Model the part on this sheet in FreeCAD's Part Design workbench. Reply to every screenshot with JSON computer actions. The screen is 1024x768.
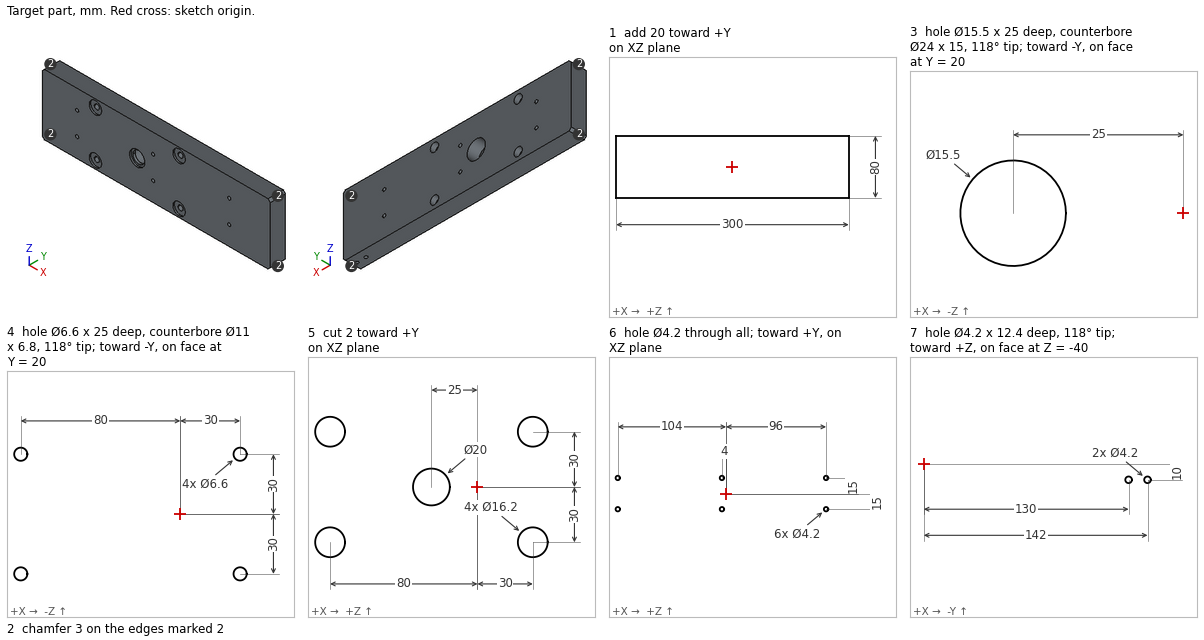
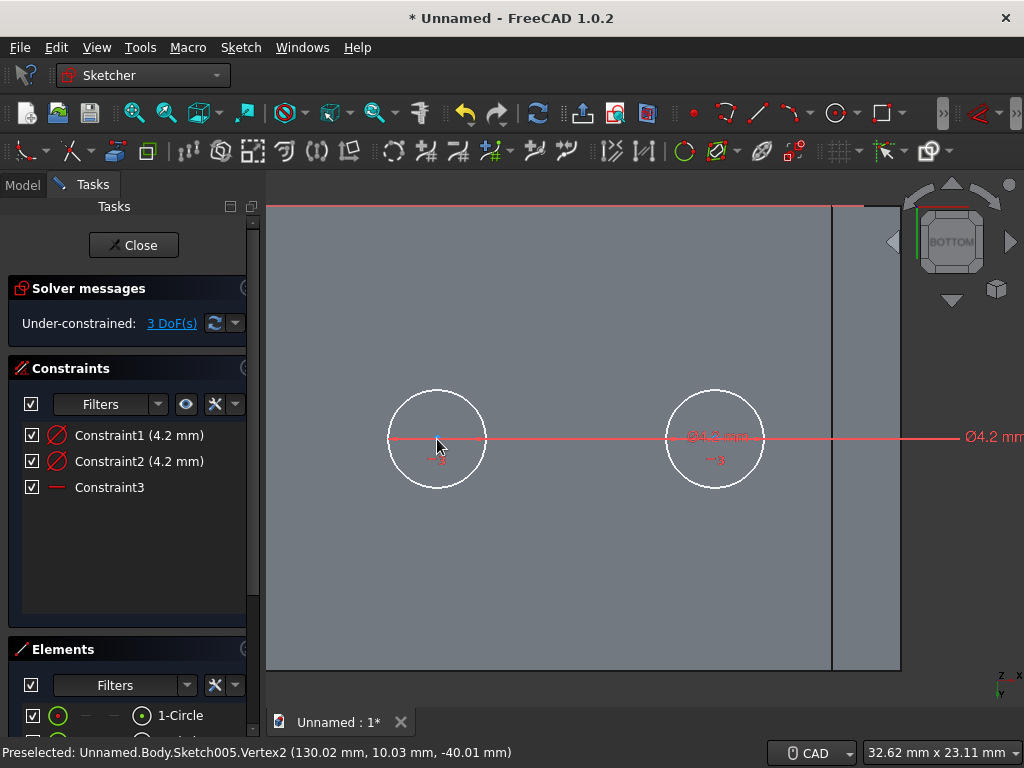
{"action": "left_click", "coordinate": [978, 114]}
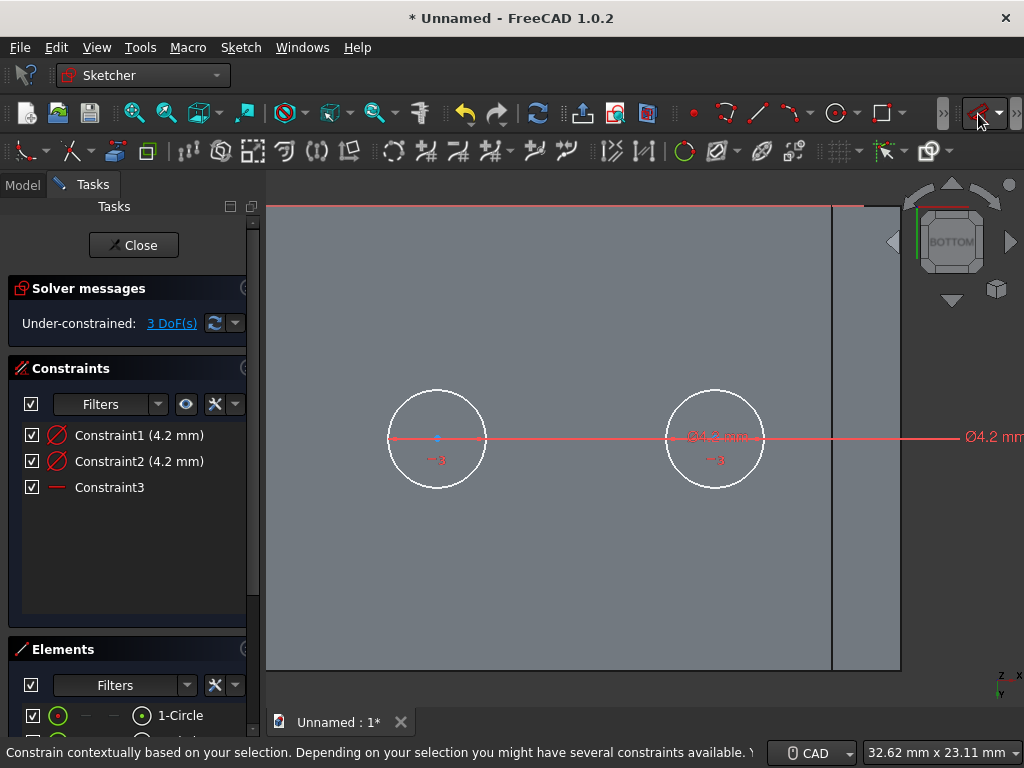
{"action": "left_click", "coordinate": [715, 439]}
{"action": "left_click", "coordinate": [749, 322]}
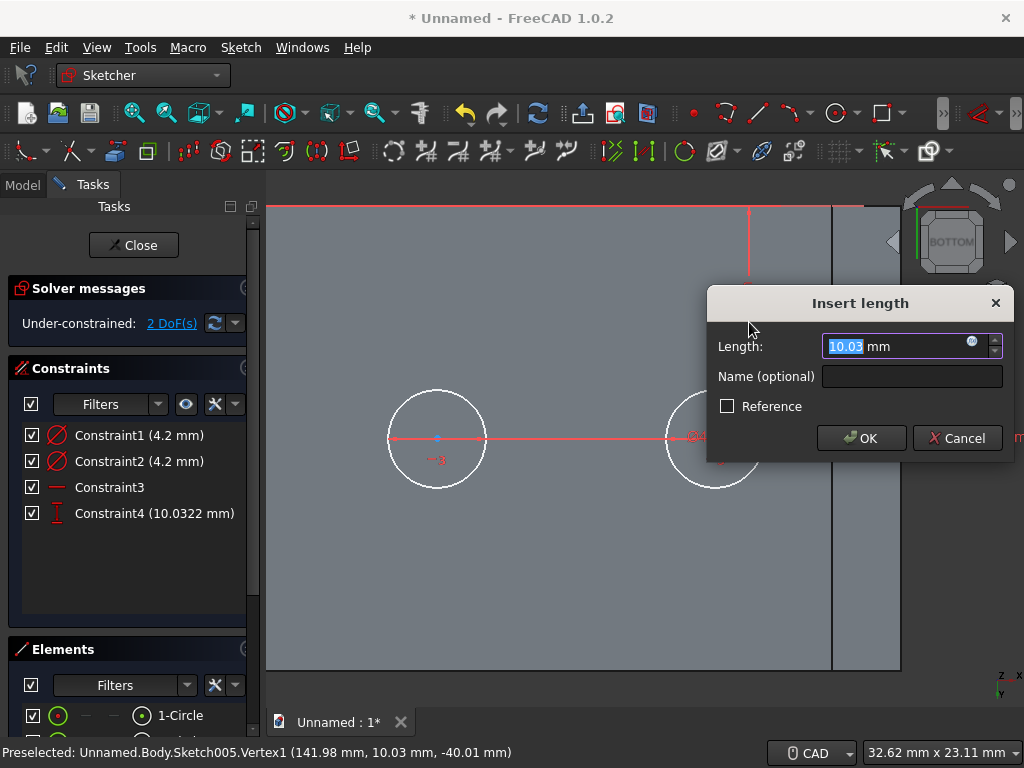
{"action": "type", "text": "10"}
{"action": "key", "text": "Return"}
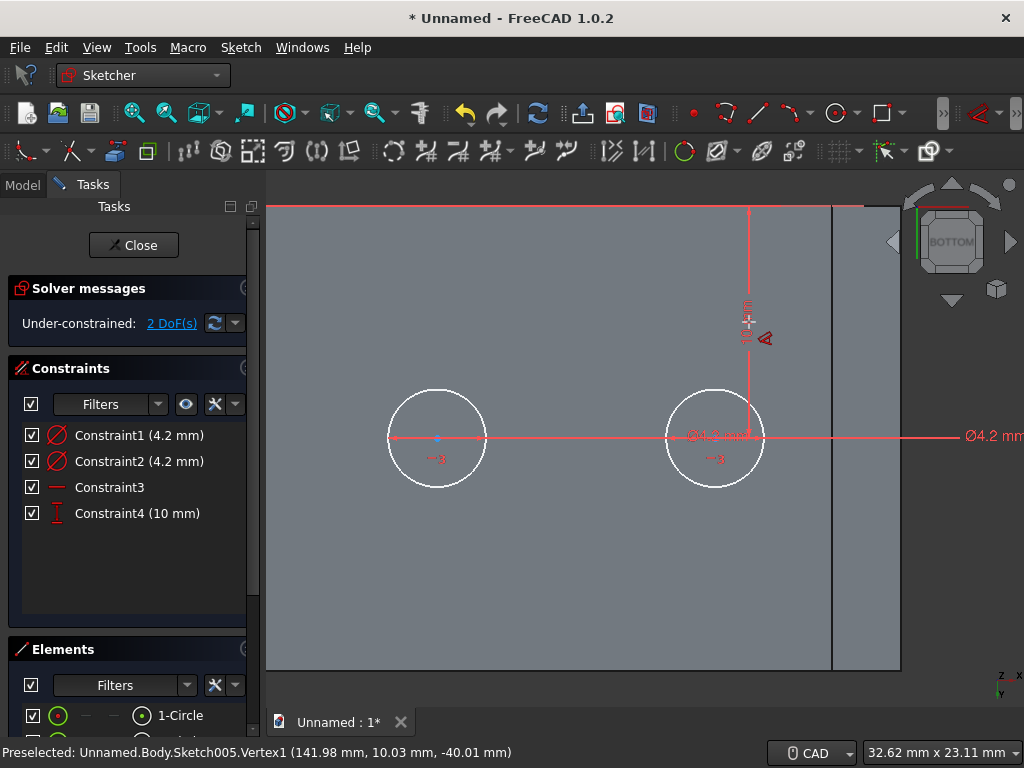
{"action": "left_click", "coordinate": [715, 438]}
{"action": "left_click", "coordinate": [504, 472]}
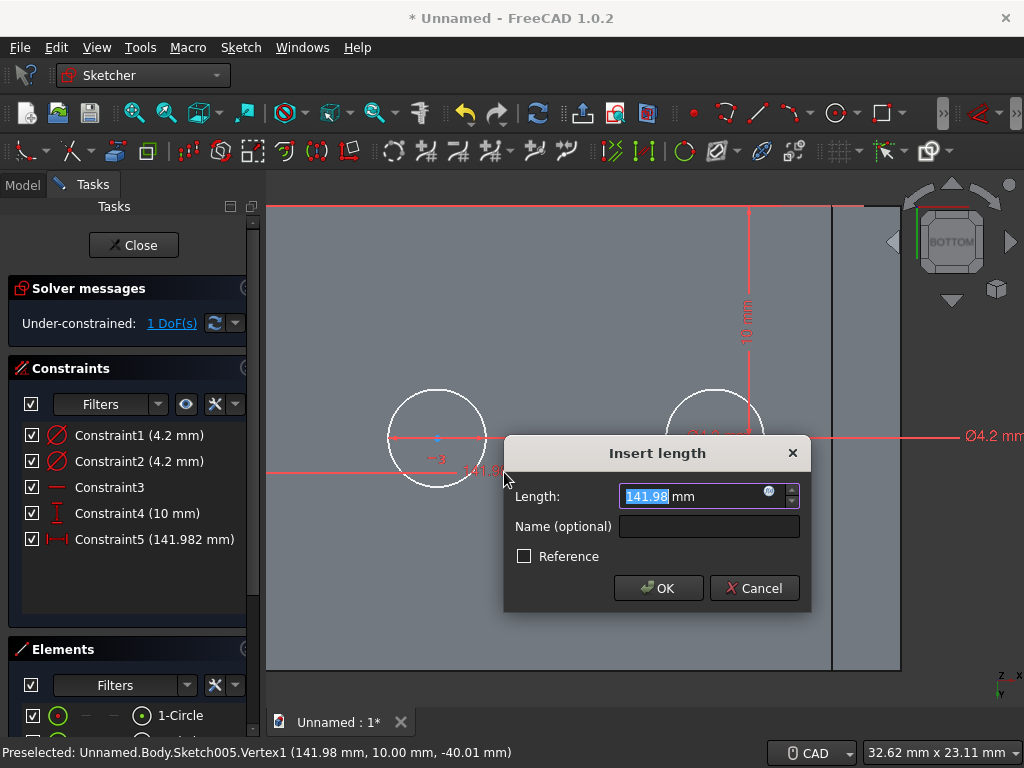
{"action": "type", "text": "142"}
{"action": "key", "text": "Return"}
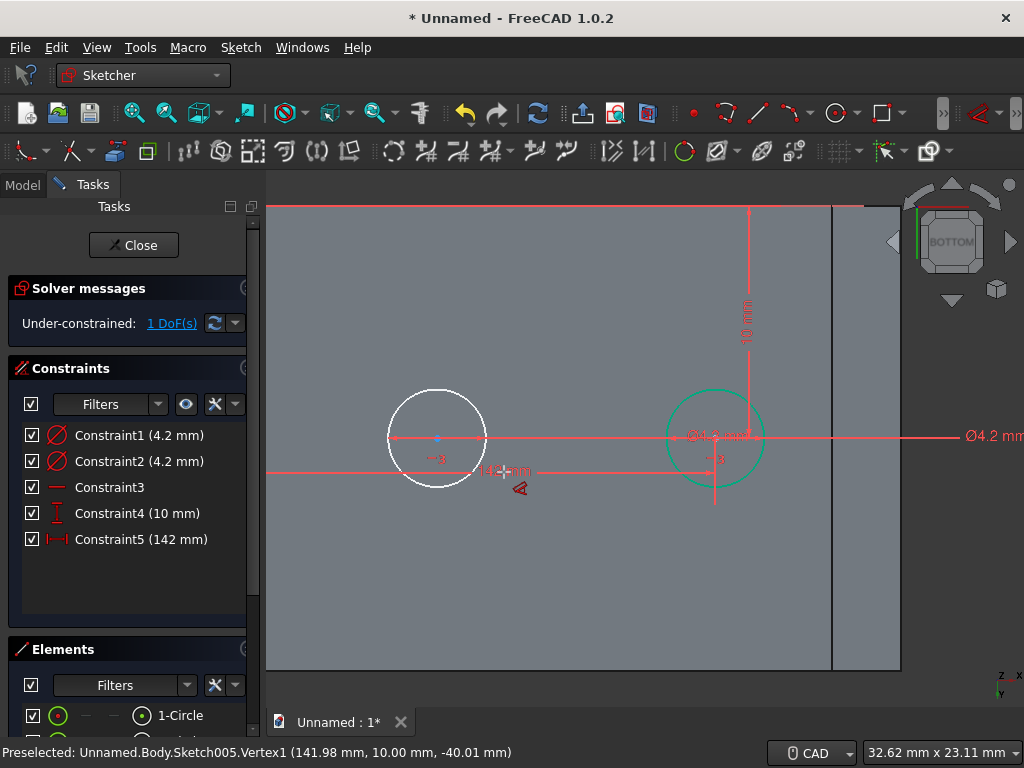
{"action": "left_click", "coordinate": [437, 438]}
{"action": "left_click", "coordinate": [365, 472]}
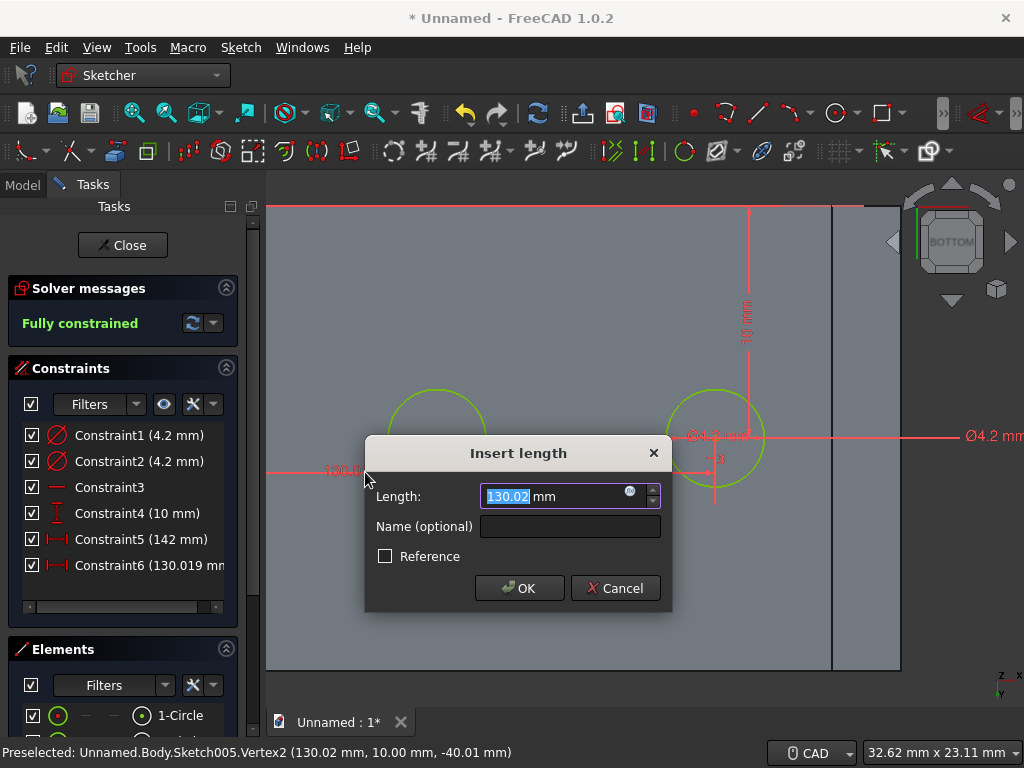
{"action": "type", "text": "130"}
{"action": "key", "text": "Return"}
{"action": "key", "text": "Escape"}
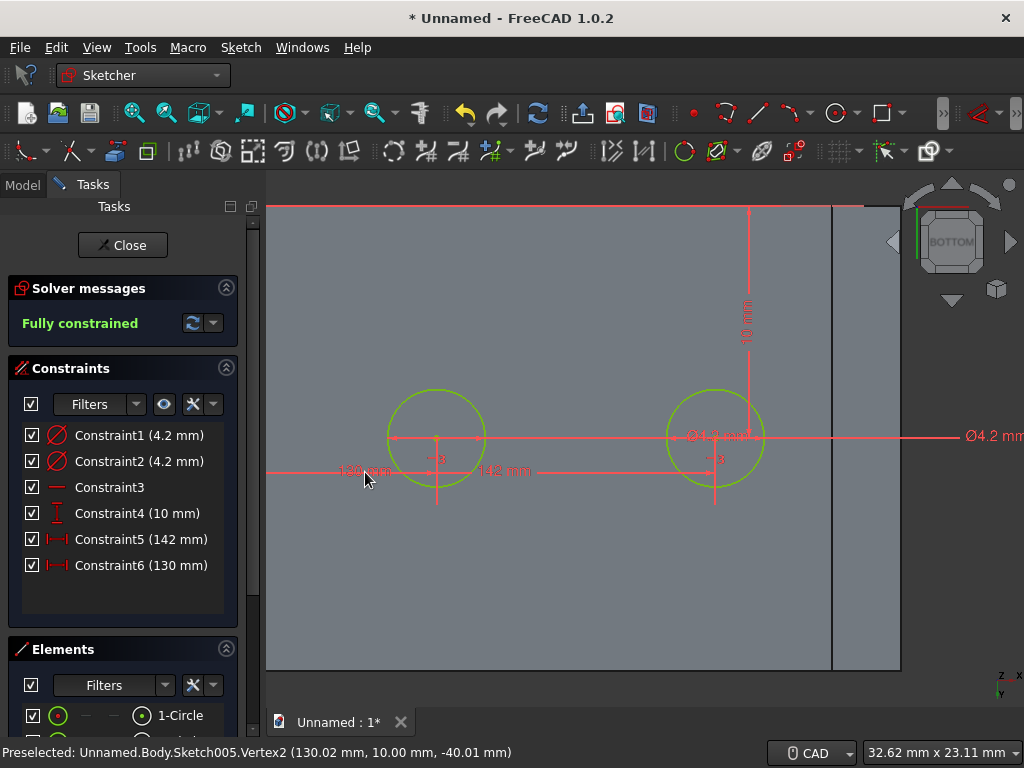
{"action": "left_click", "coordinate": [123, 245]}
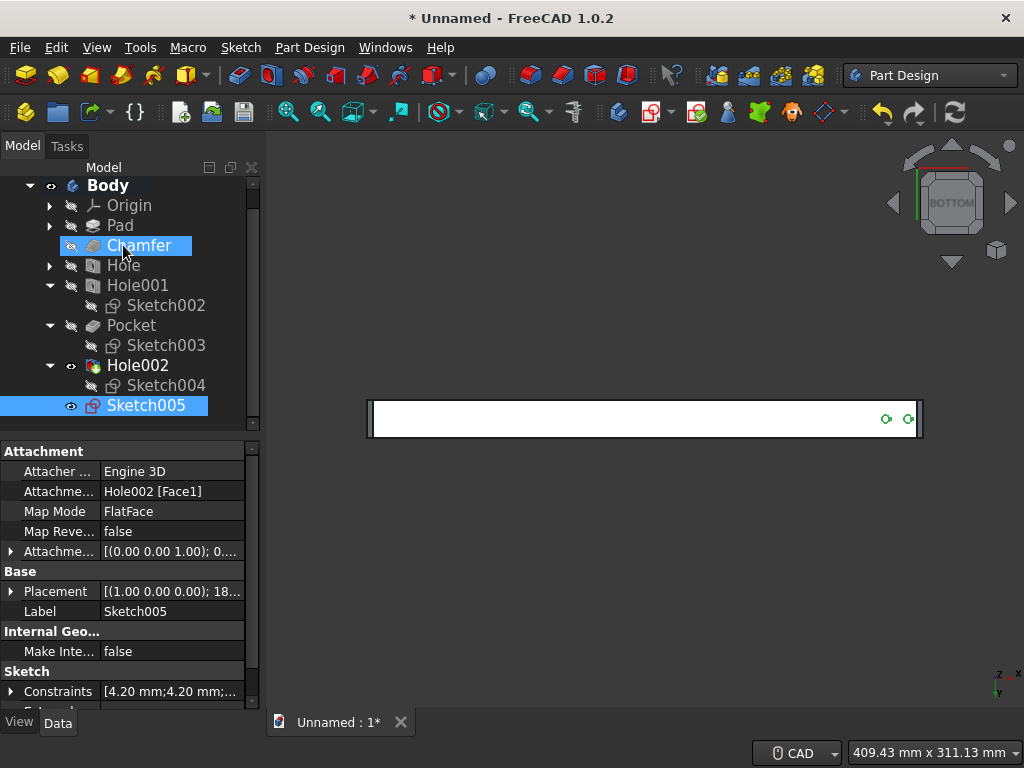
{"action": "left_click", "coordinate": [272, 76]}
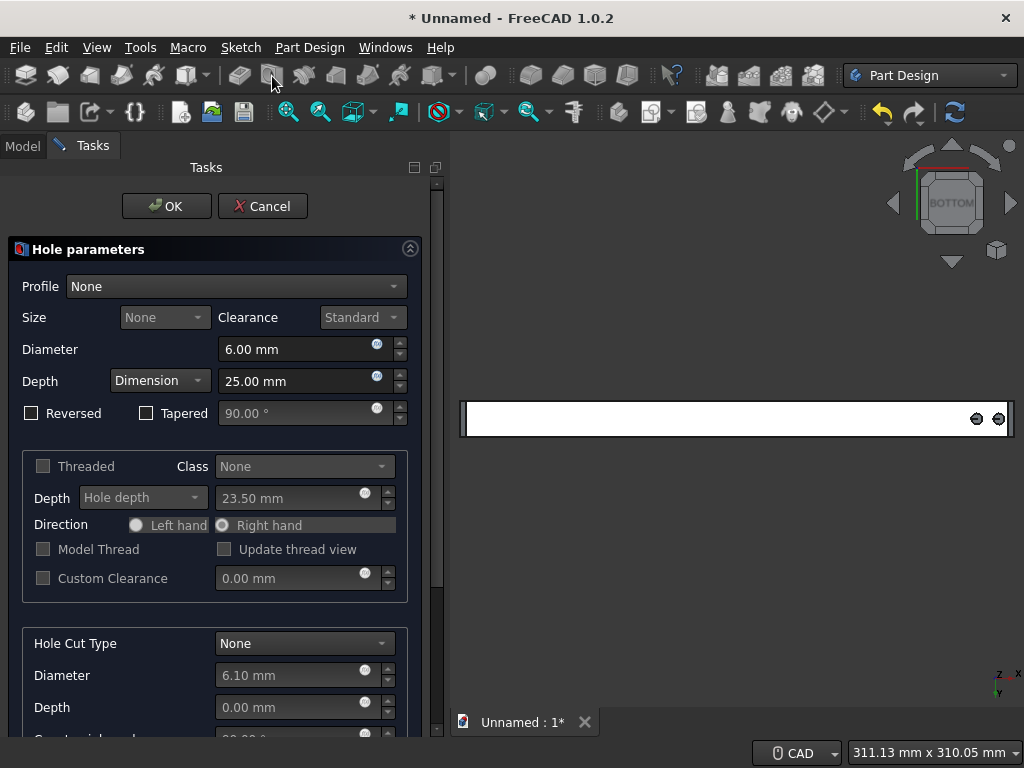
{"action": "triple_click", "coordinate": [305, 349]}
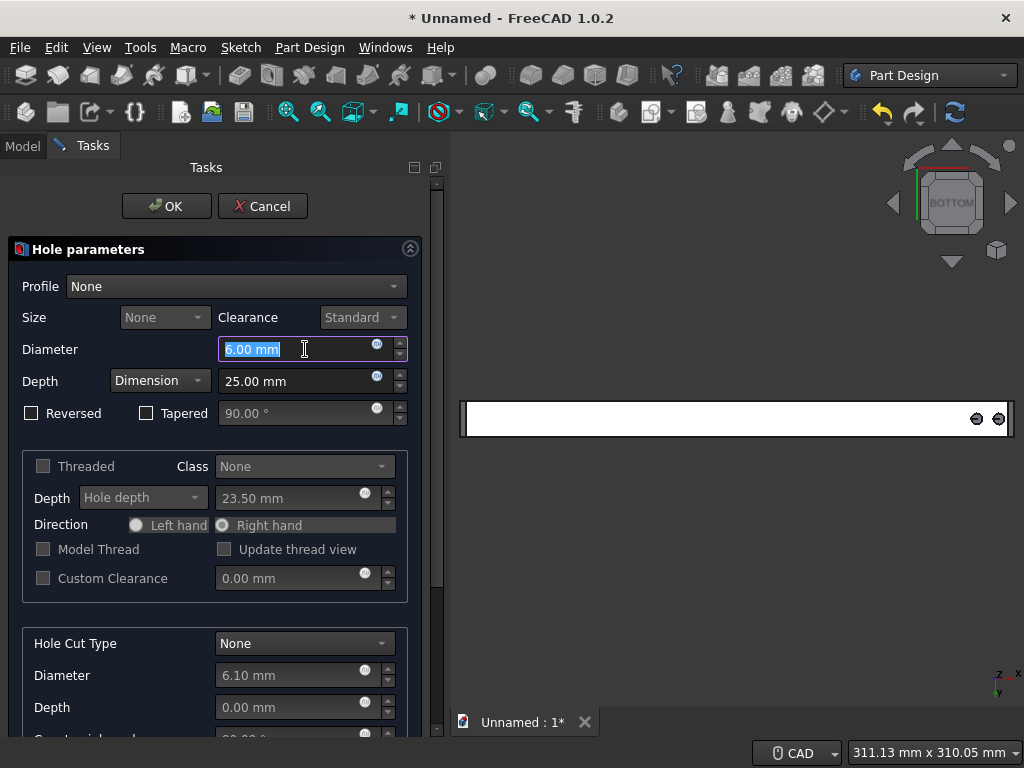
{"action": "type", "text": "4.2"}
{"action": "key", "text": "Tab"}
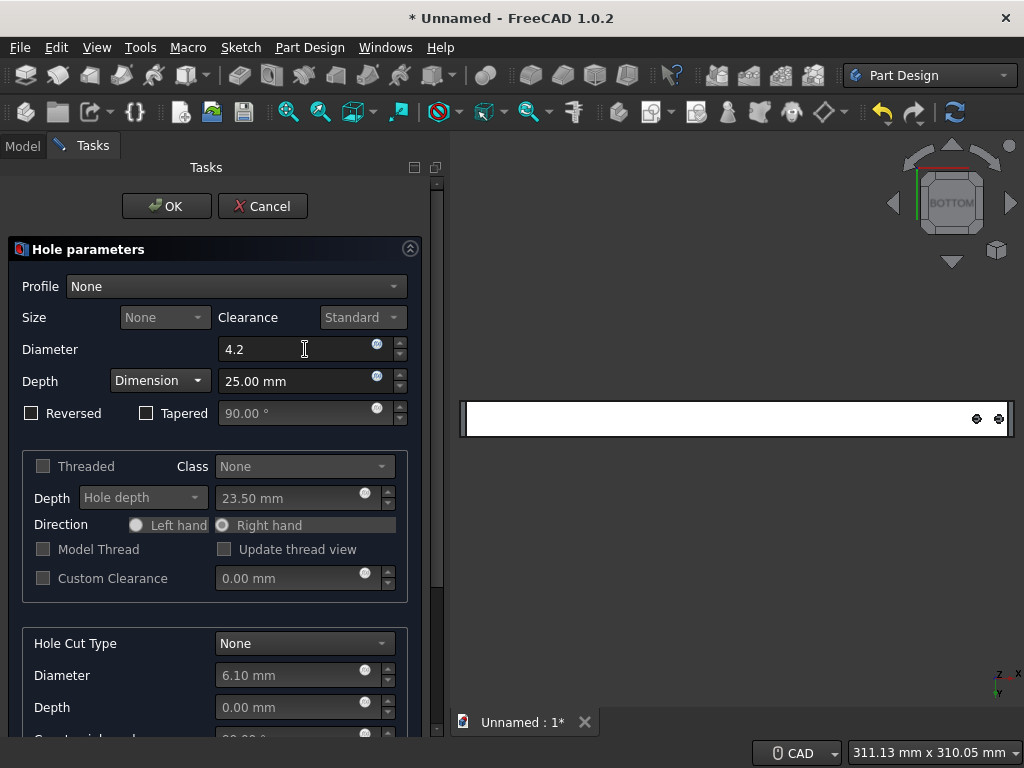
{"action": "triple_click", "coordinate": [305, 381]}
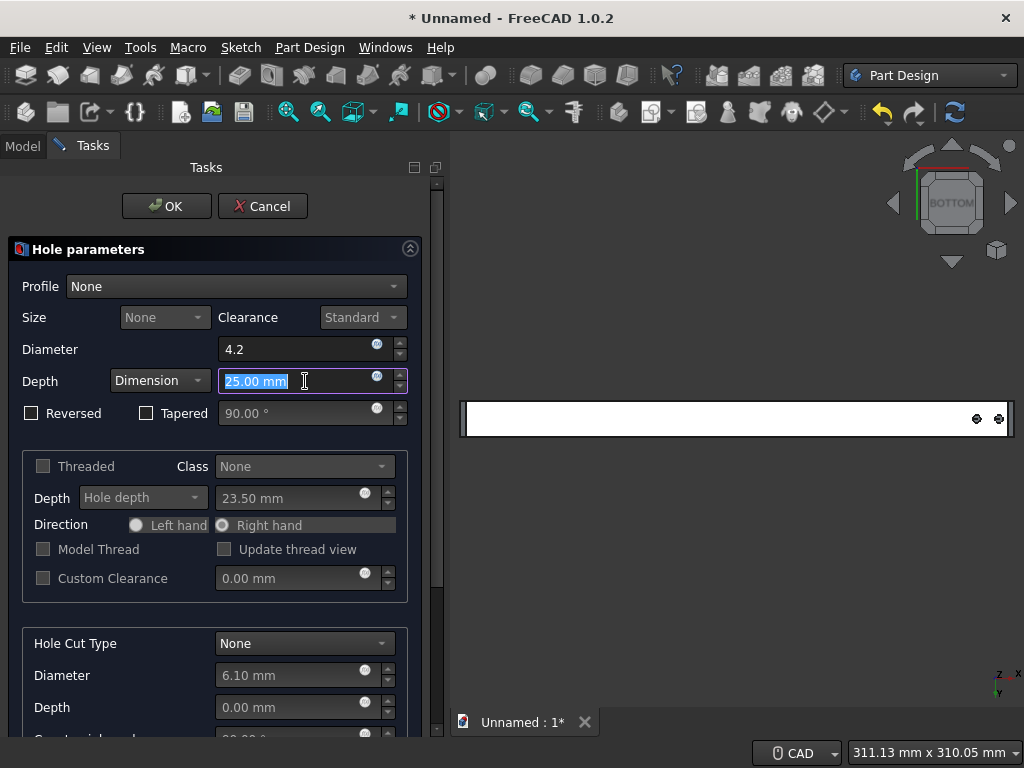
{"action": "type", "text": "12.4"}
{"action": "key", "text": "Tab"}